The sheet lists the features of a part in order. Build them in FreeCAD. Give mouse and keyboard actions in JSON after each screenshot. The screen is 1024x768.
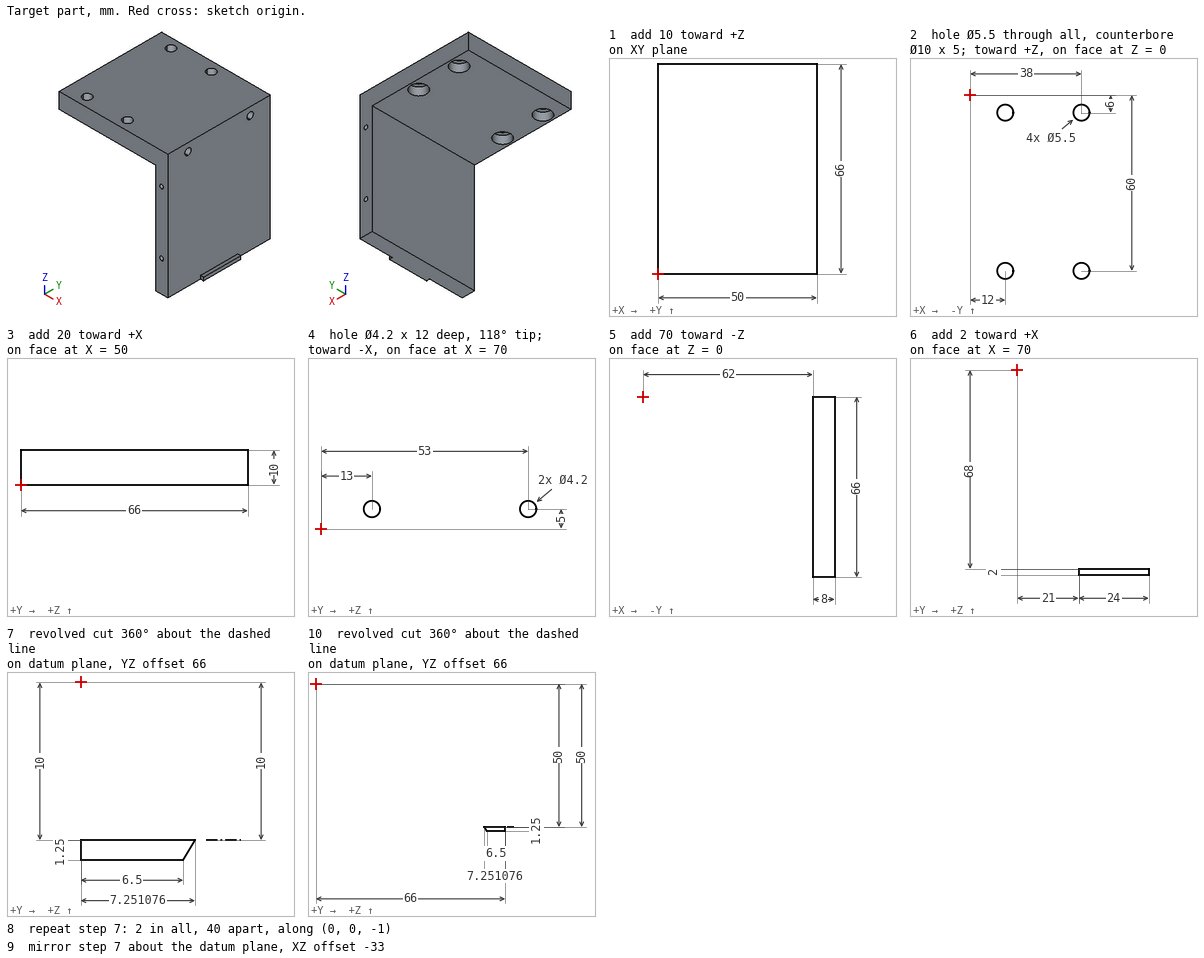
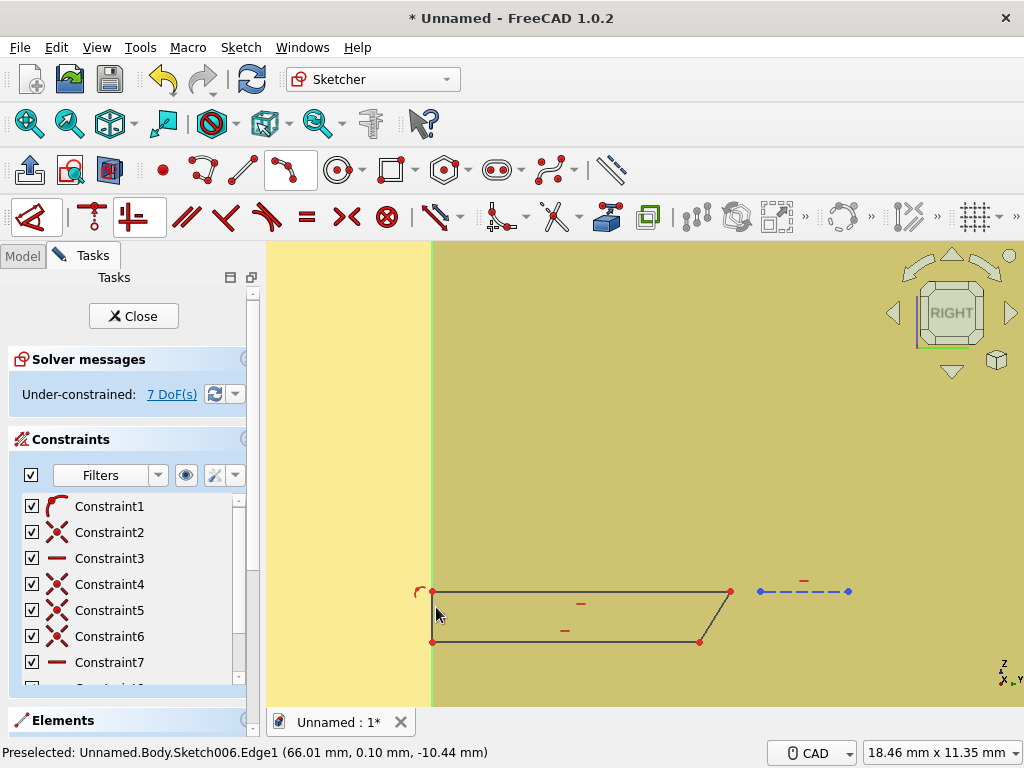
{"action": "left_click", "coordinate": [513, 642]}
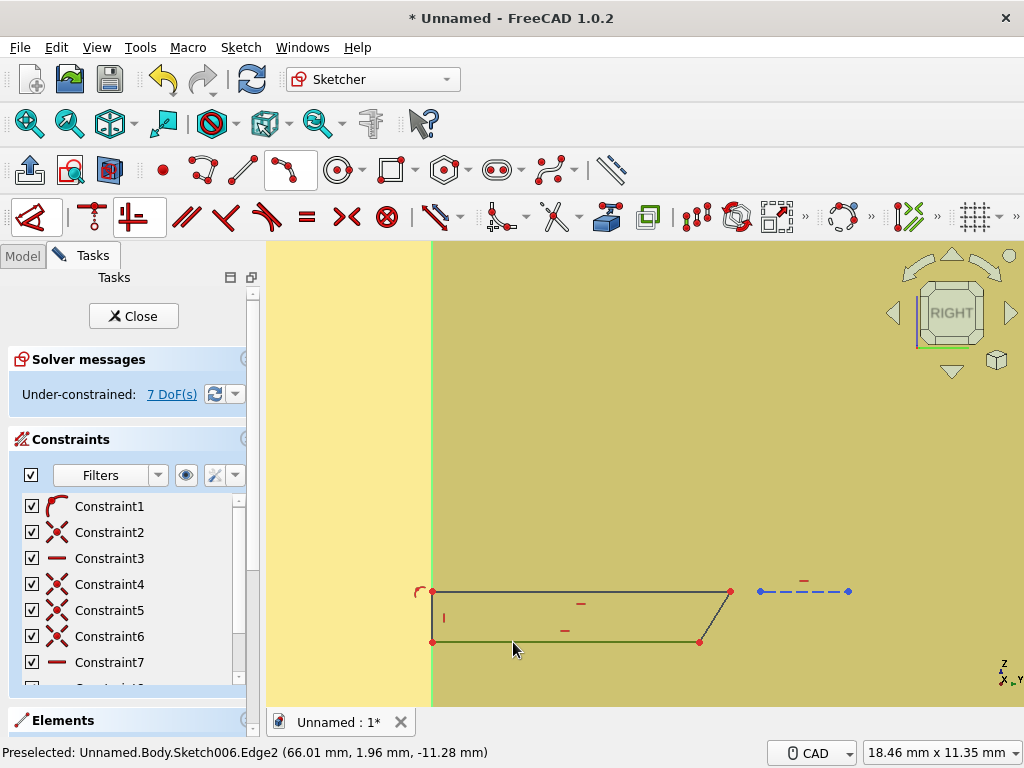
{"action": "key", "text": "l"}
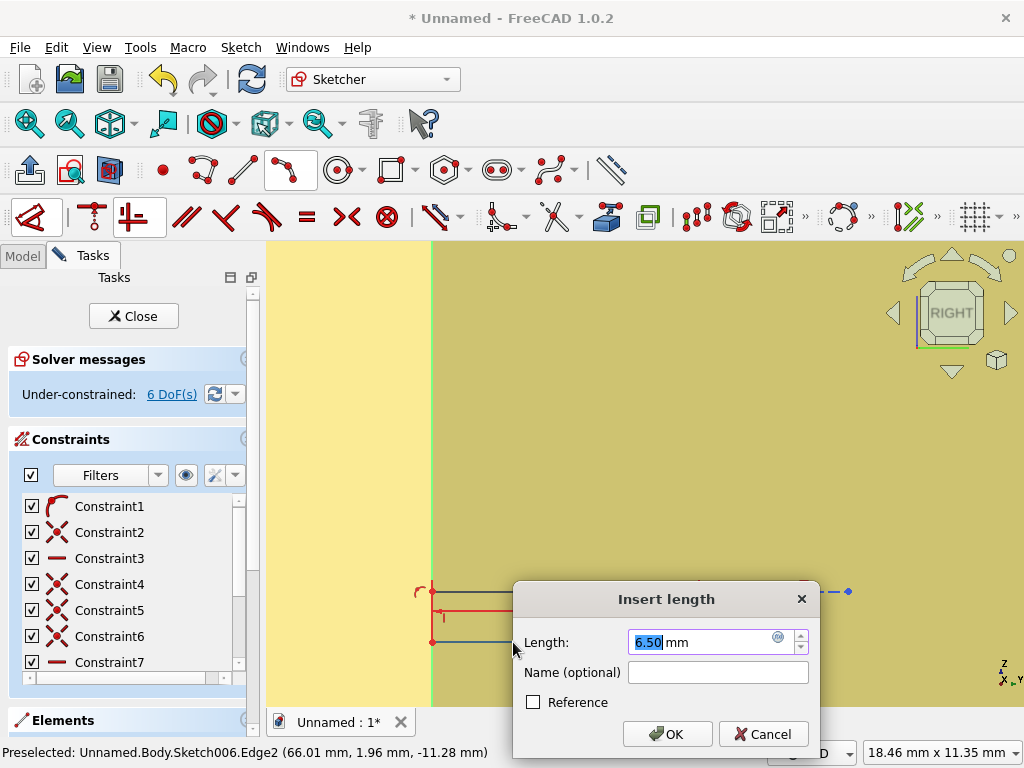
{"action": "type", "text": "6.5"}
{"action": "key", "text": "Return"}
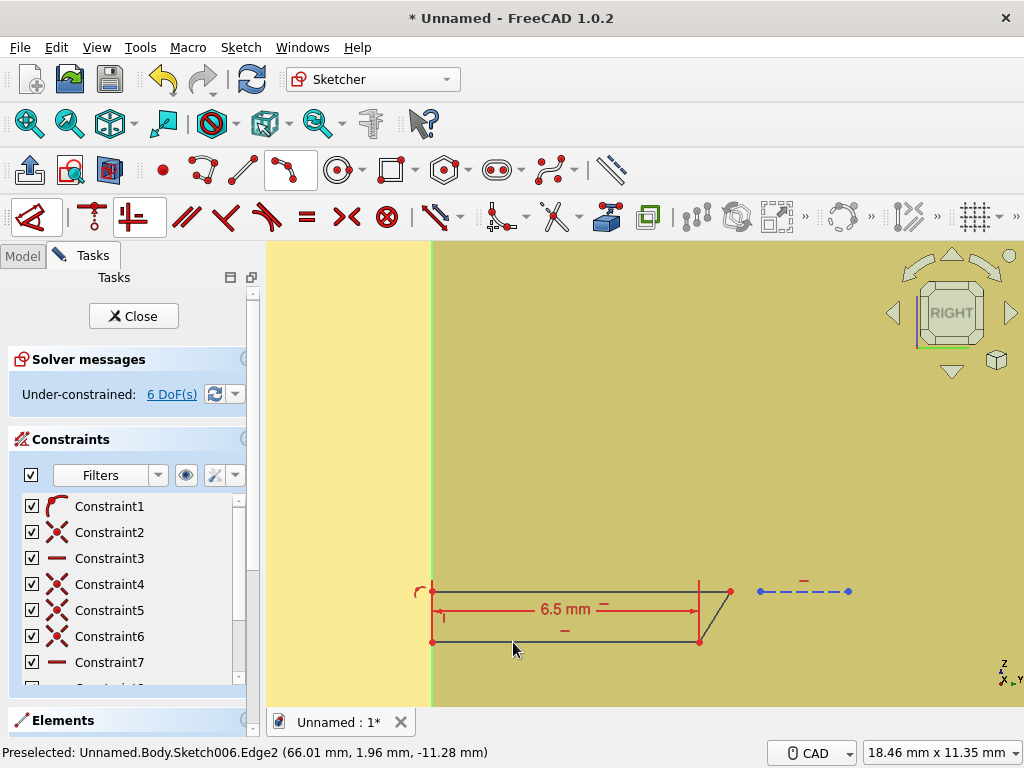
{"action": "left_click", "coordinate": [432, 592]}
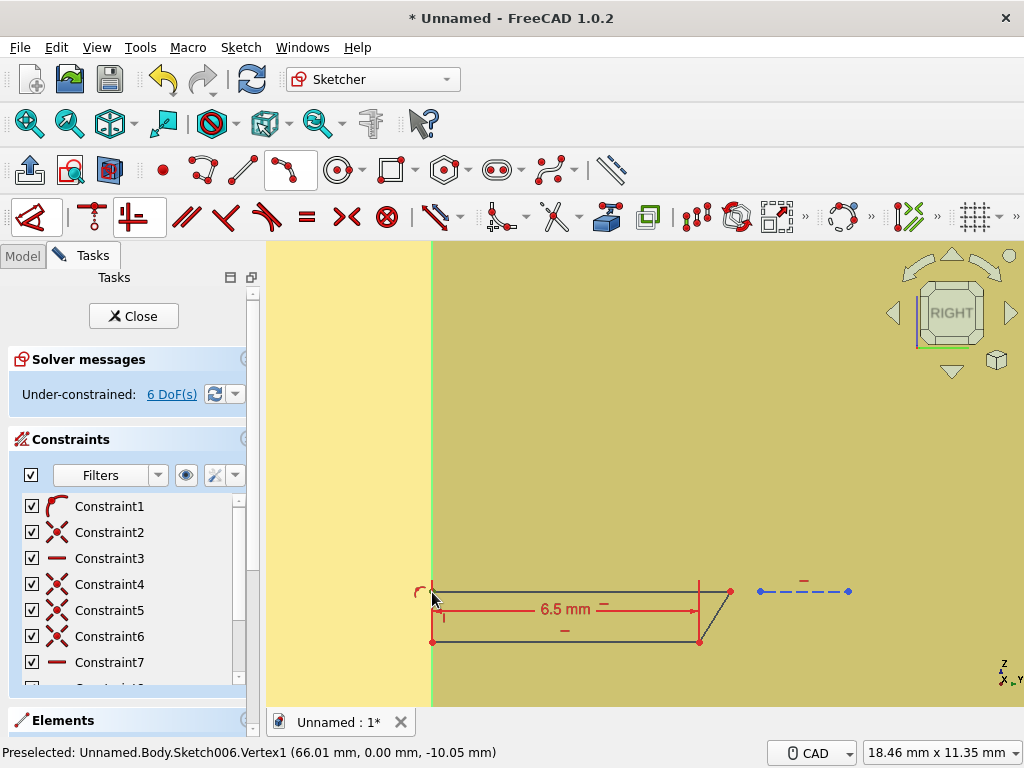
{"action": "key", "text": "i"}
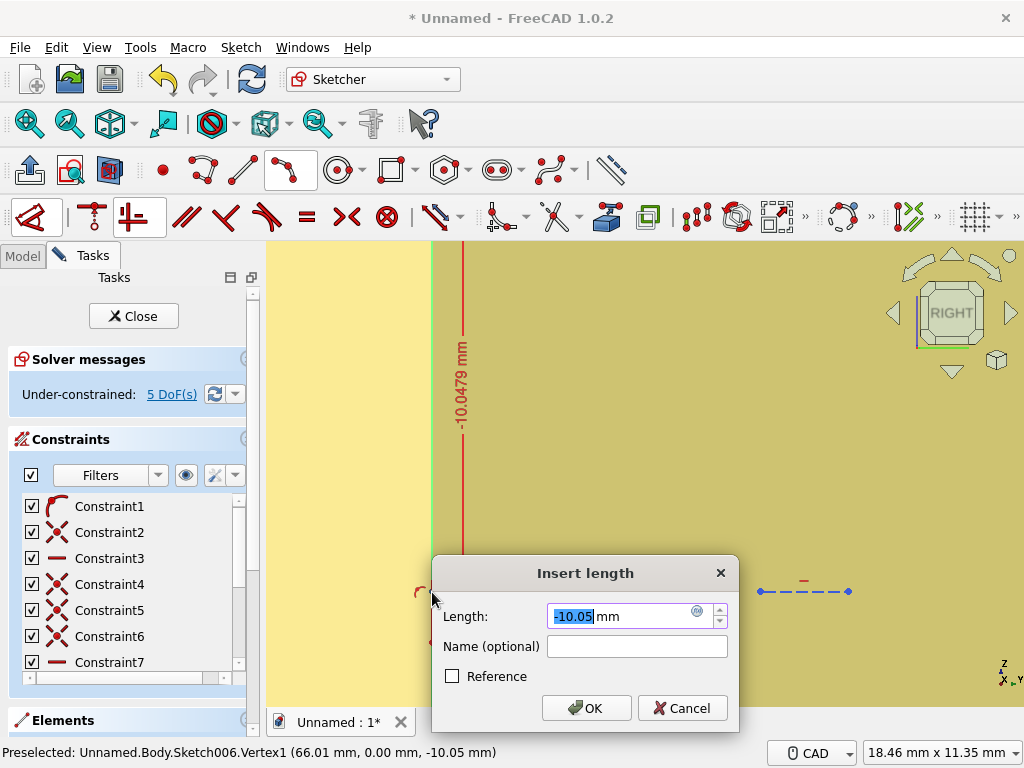
{"action": "type", "text": "-10"}
{"action": "key", "text": "Return"}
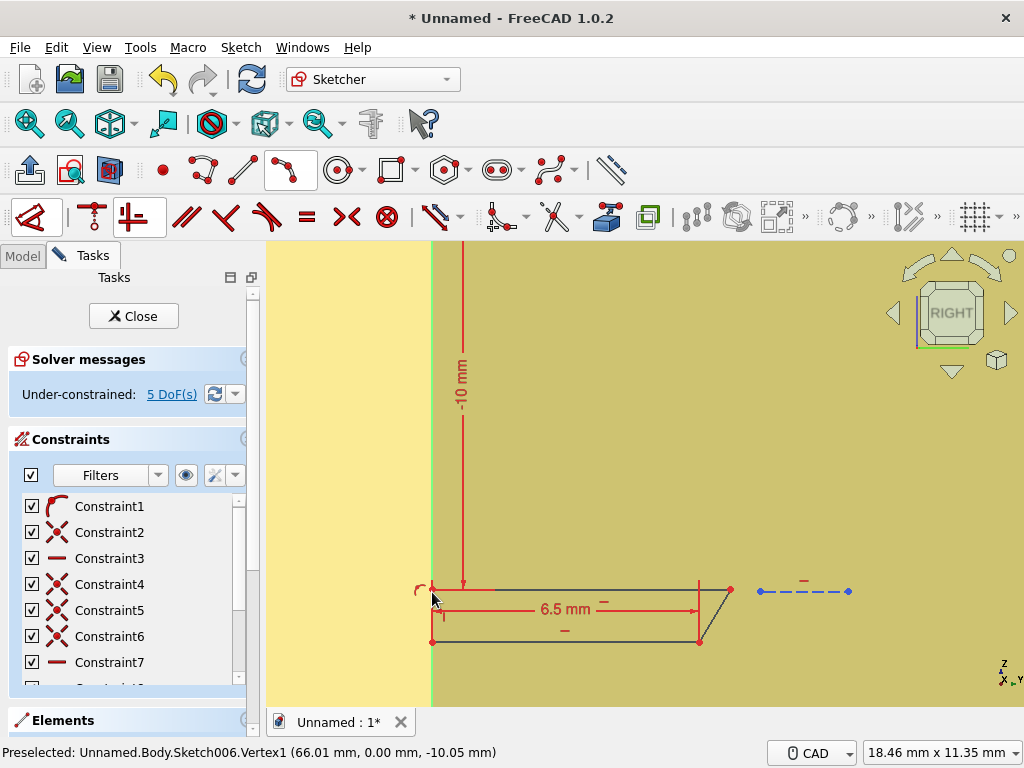
{"action": "left_click", "coordinate": [761, 592]}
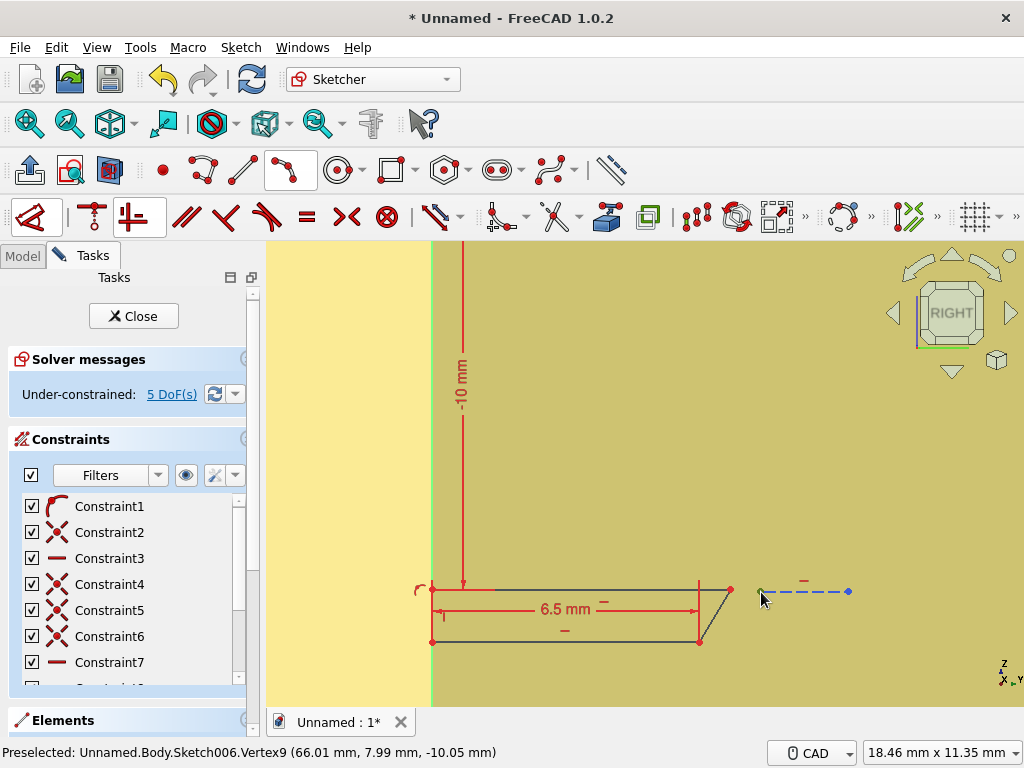
{"action": "key", "text": "i"}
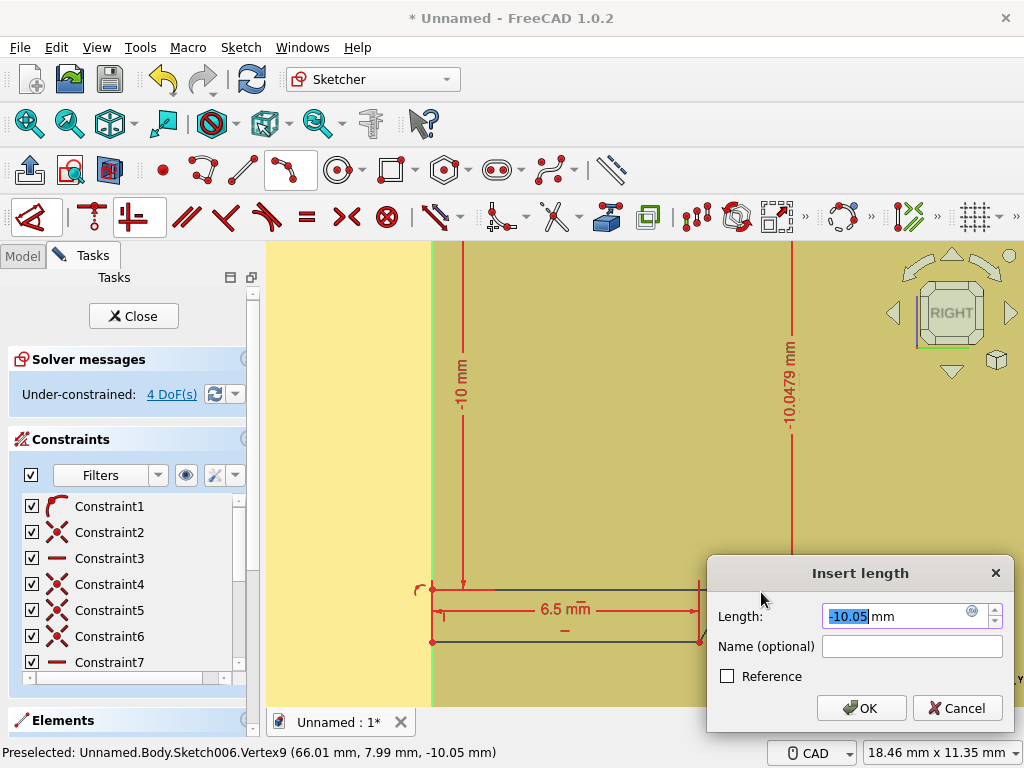
{"action": "type", "text": "-10"}
{"action": "key", "text": "Return"}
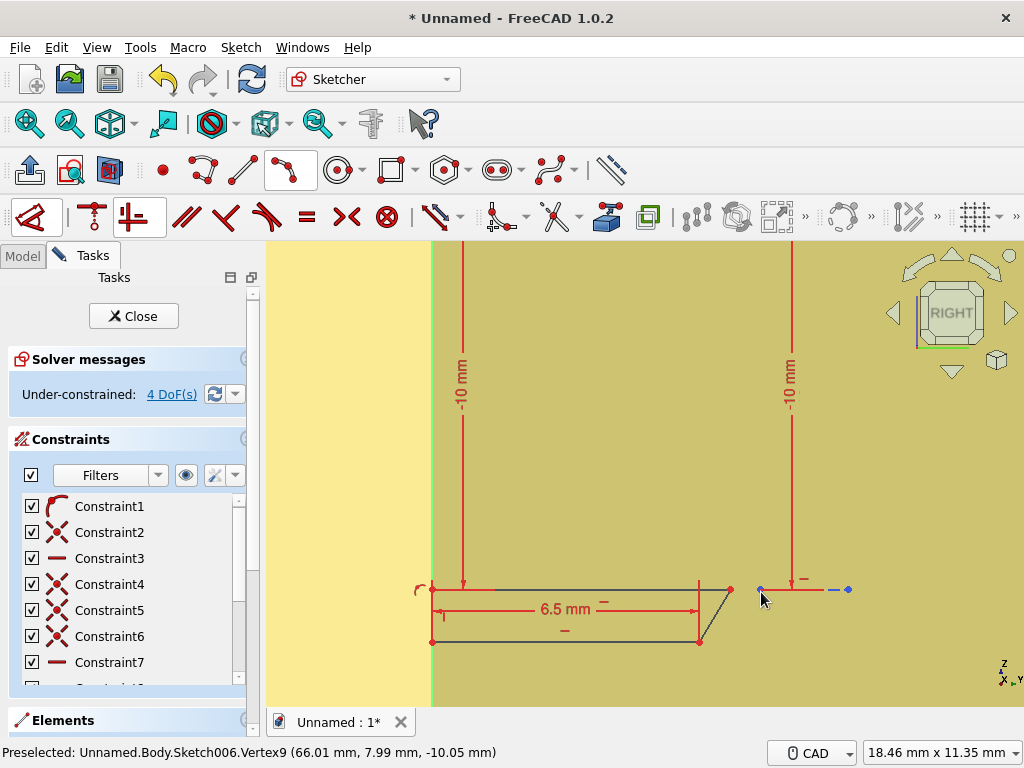
{"action": "left_click", "coordinate": [432, 606]}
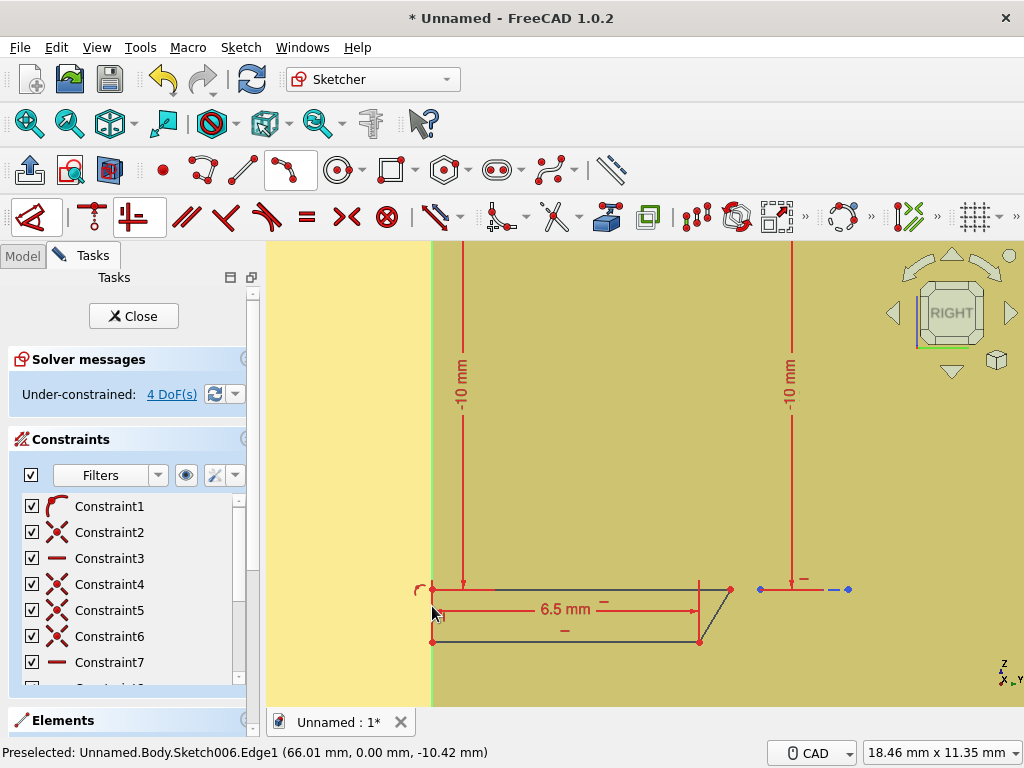
{"action": "key", "text": "i"}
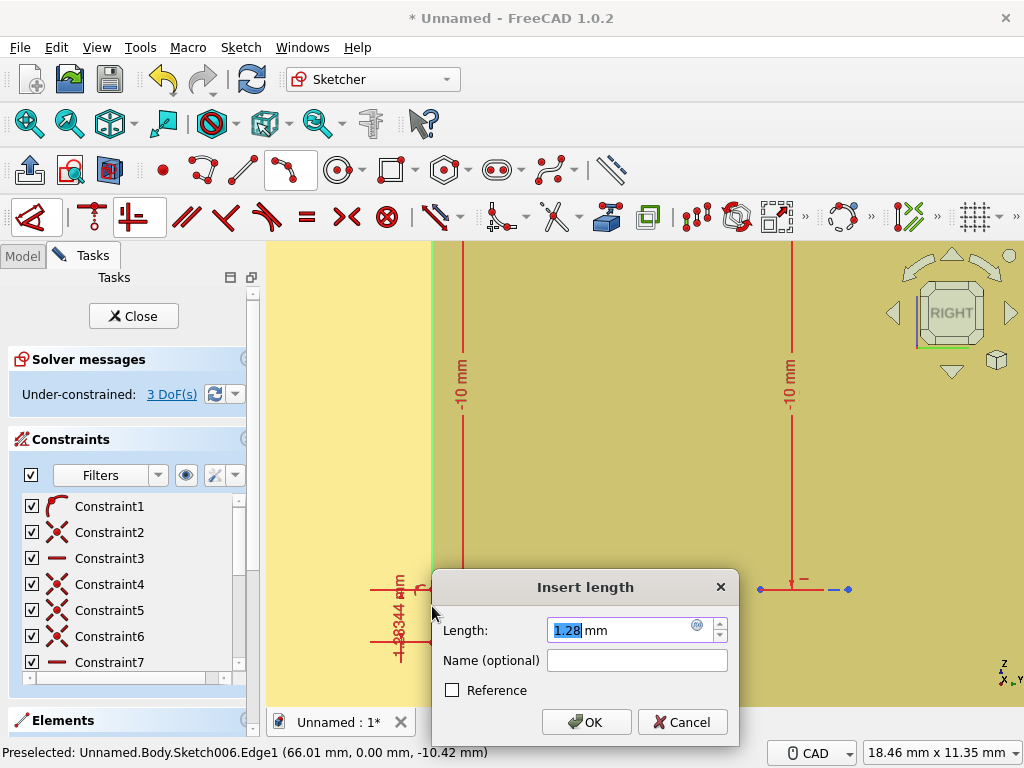
{"action": "type", "text": "1.25"}
{"action": "key", "text": "Return"}